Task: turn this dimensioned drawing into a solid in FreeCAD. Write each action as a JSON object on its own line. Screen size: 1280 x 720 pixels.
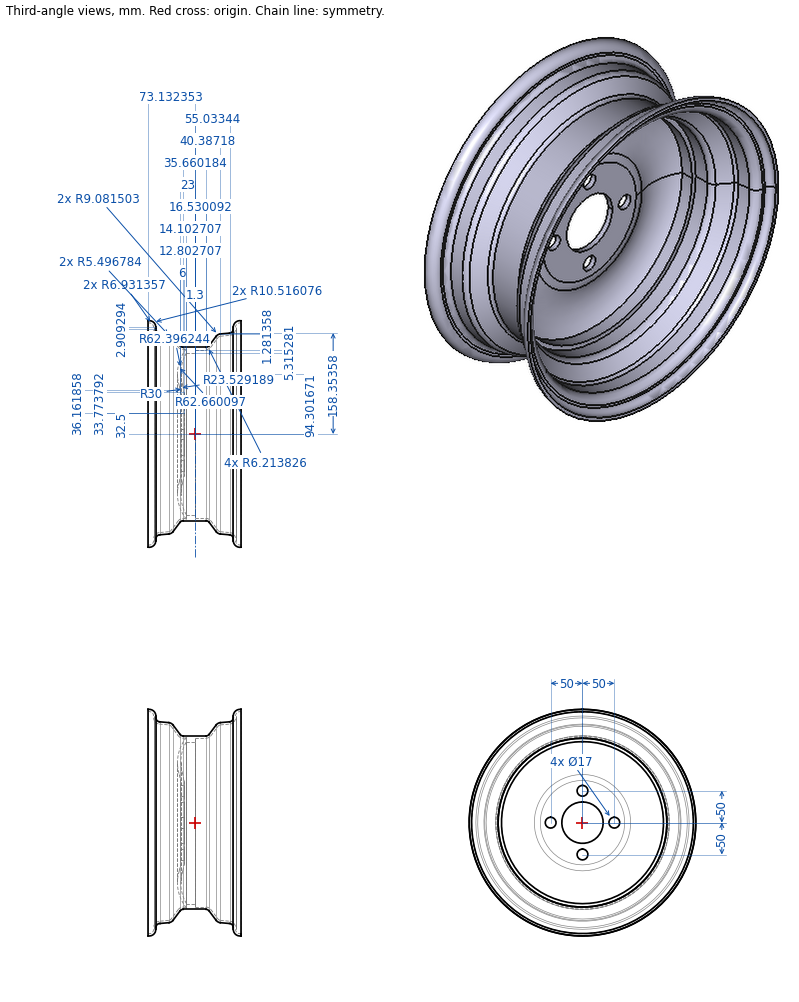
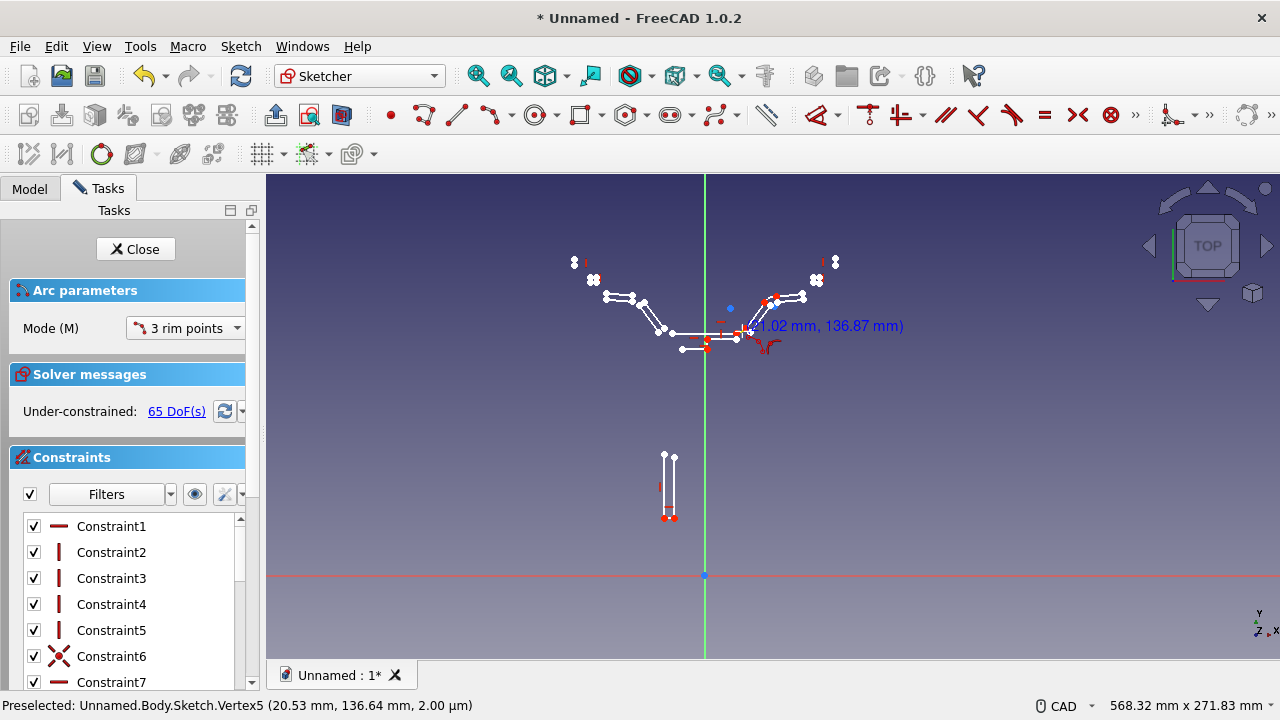
{"action": "scroll", "coordinate": [673, 333], "scroll_direction": "up", "scroll_amount": 3}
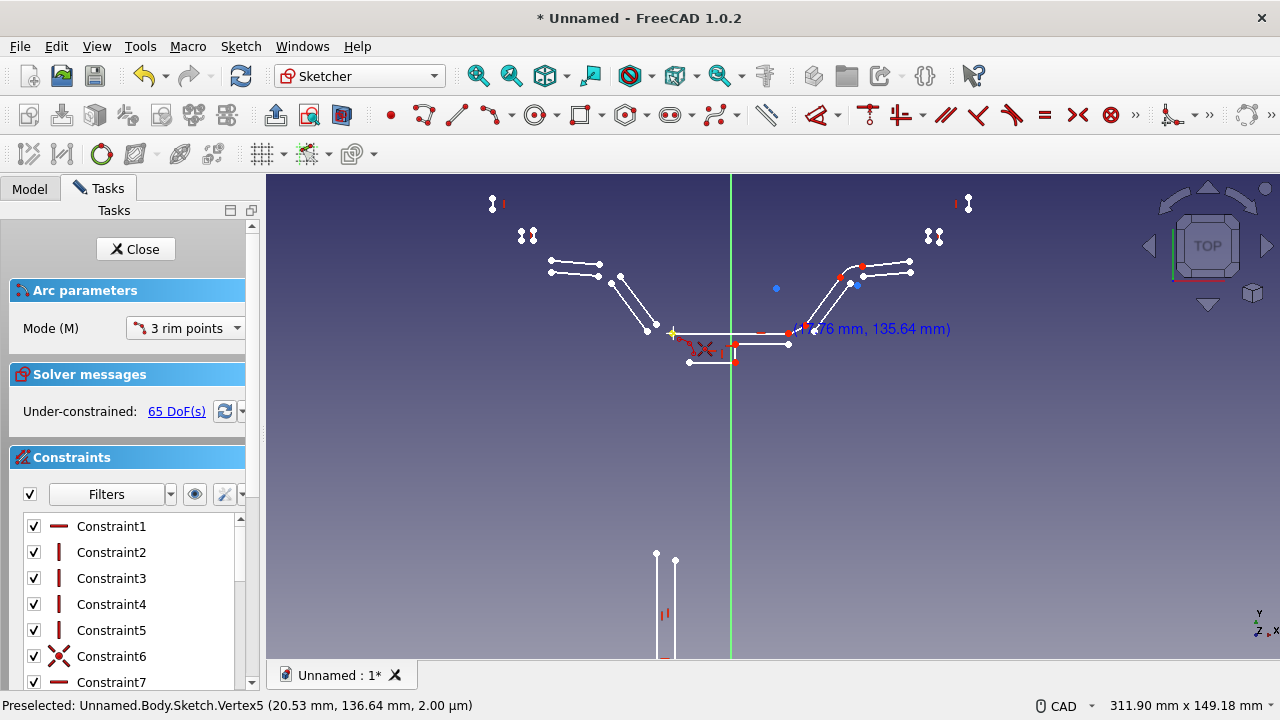
{"action": "left_click", "coordinate": [673, 334]}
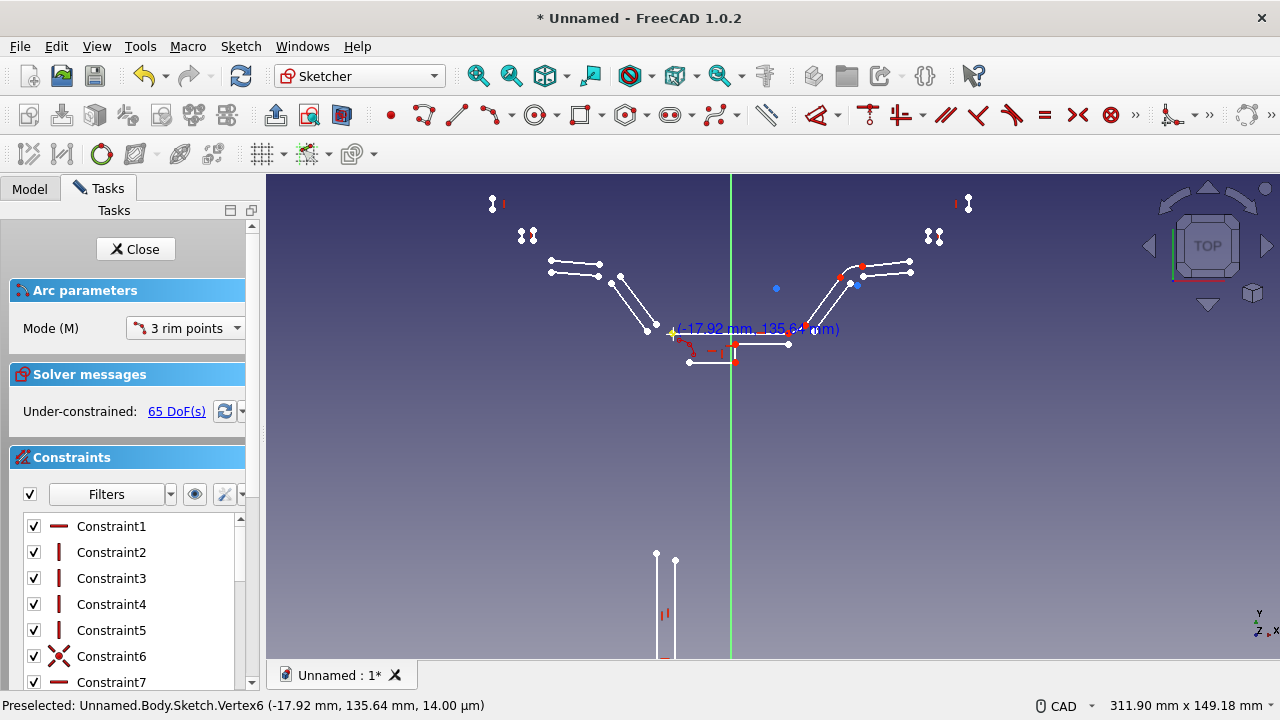
{"action": "scroll", "coordinate": [657, 324], "scroll_direction": "up", "scroll_amount": 2}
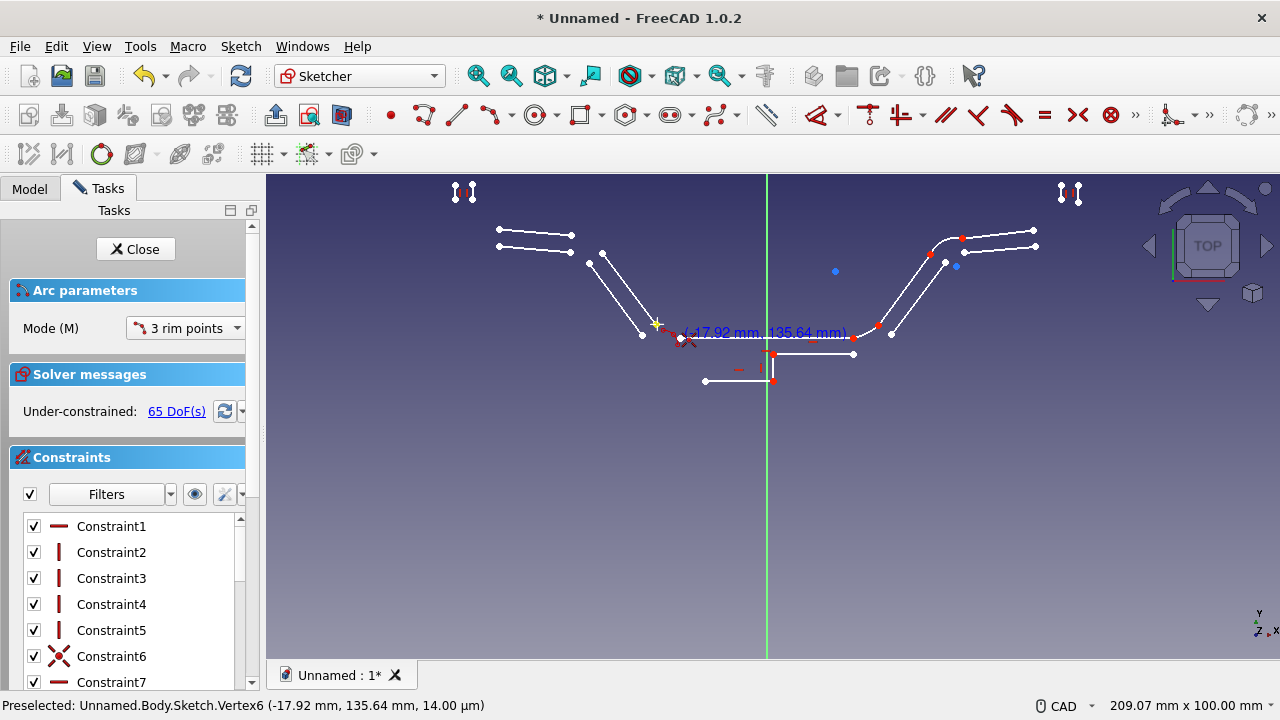
{"action": "left_click", "coordinate": [656, 325]}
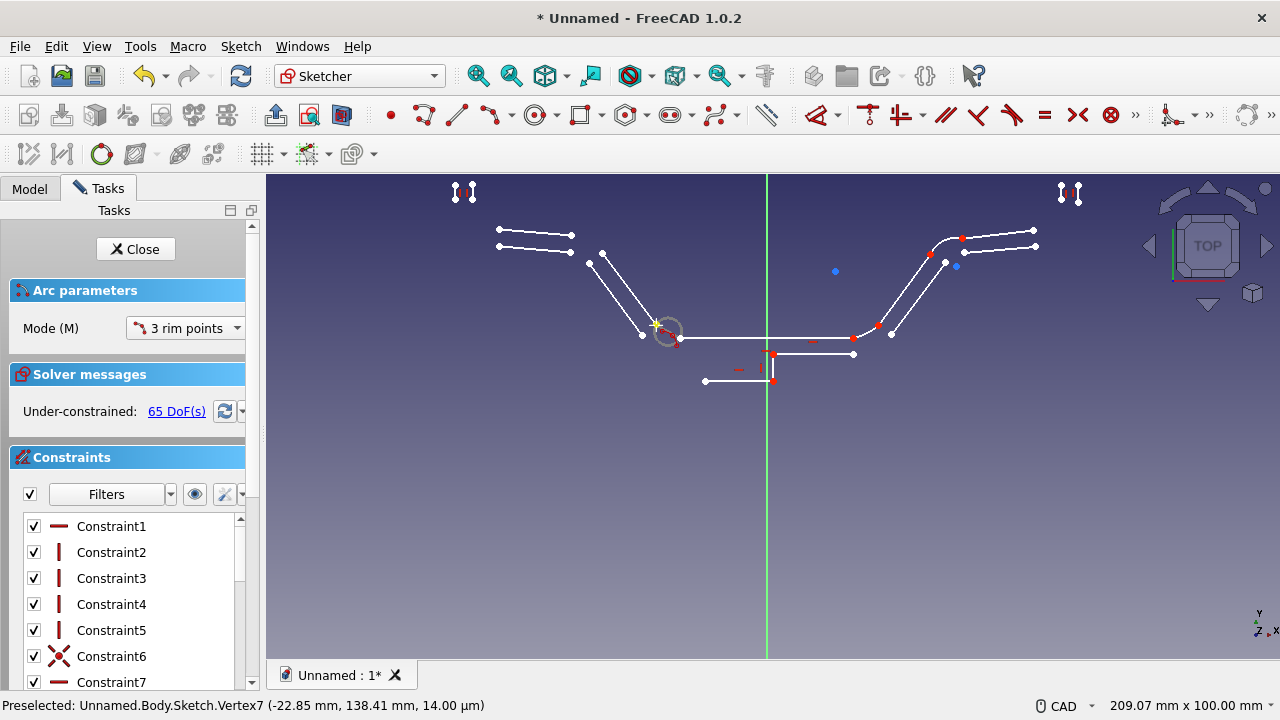
{"action": "scroll", "coordinate": [667, 333], "scroll_direction": "up", "scroll_amount": 9}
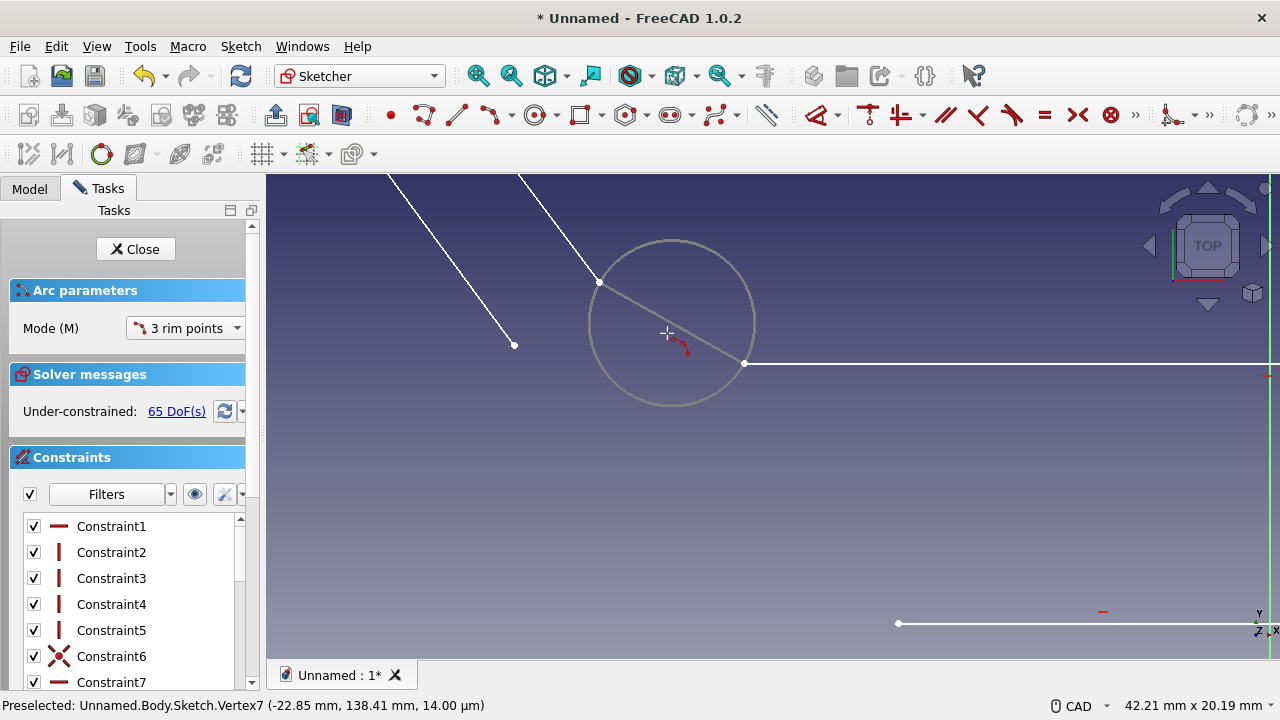
{"action": "left_click", "coordinate": [665, 331]}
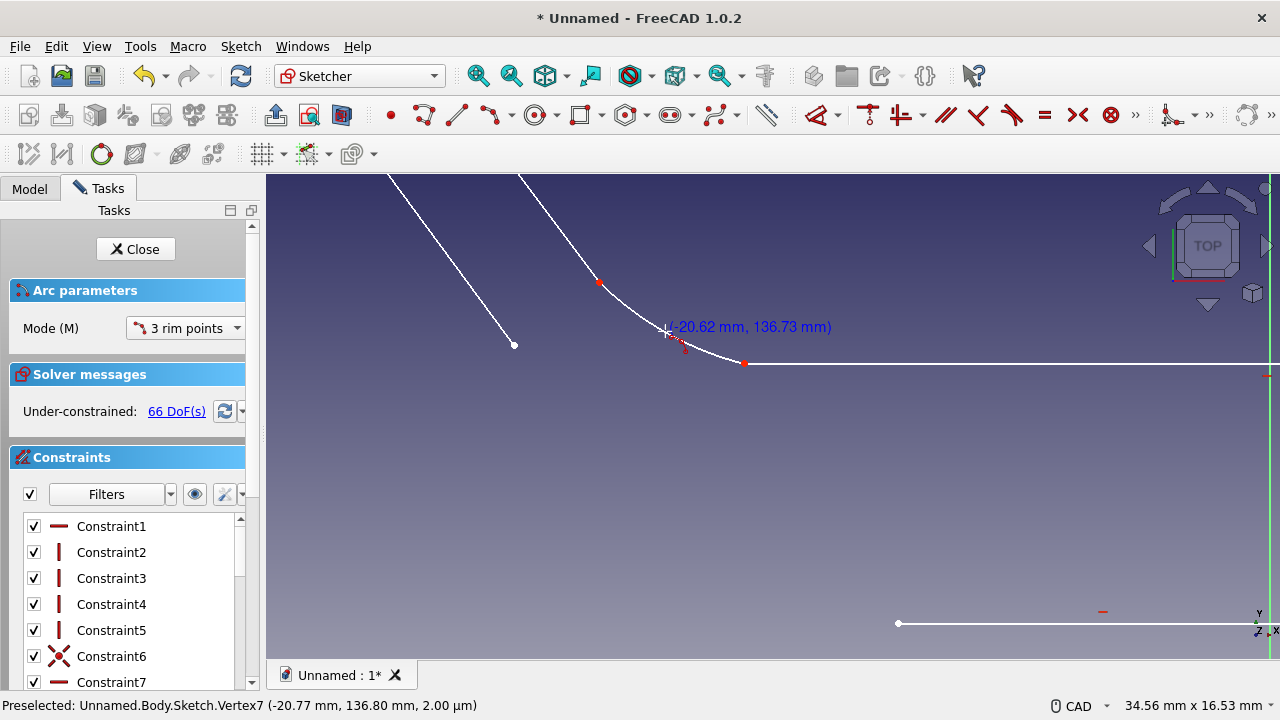
{"action": "scroll", "coordinate": [668, 331], "scroll_direction": "down", "scroll_amount": 14}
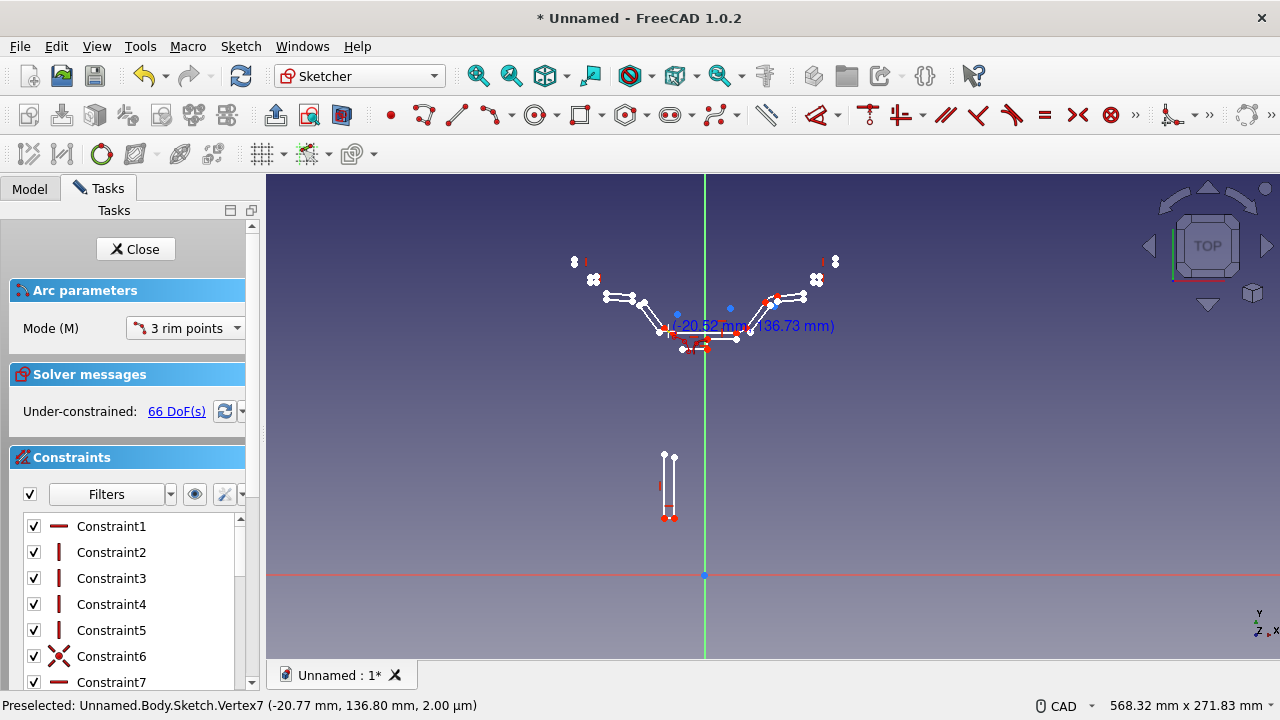
{"action": "scroll", "coordinate": [644, 302], "scroll_direction": "up", "scroll_amount": 5}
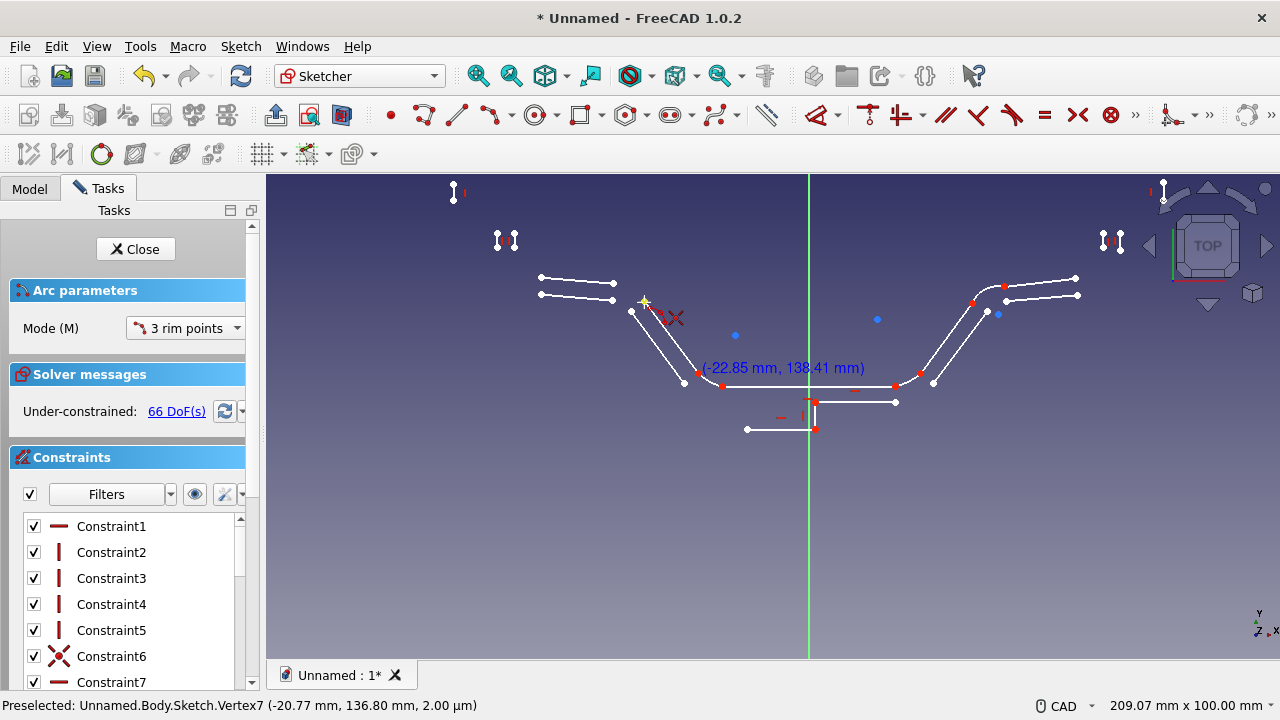
{"action": "left_click", "coordinate": [645, 302]}
{"action": "left_click", "coordinate": [613, 284]}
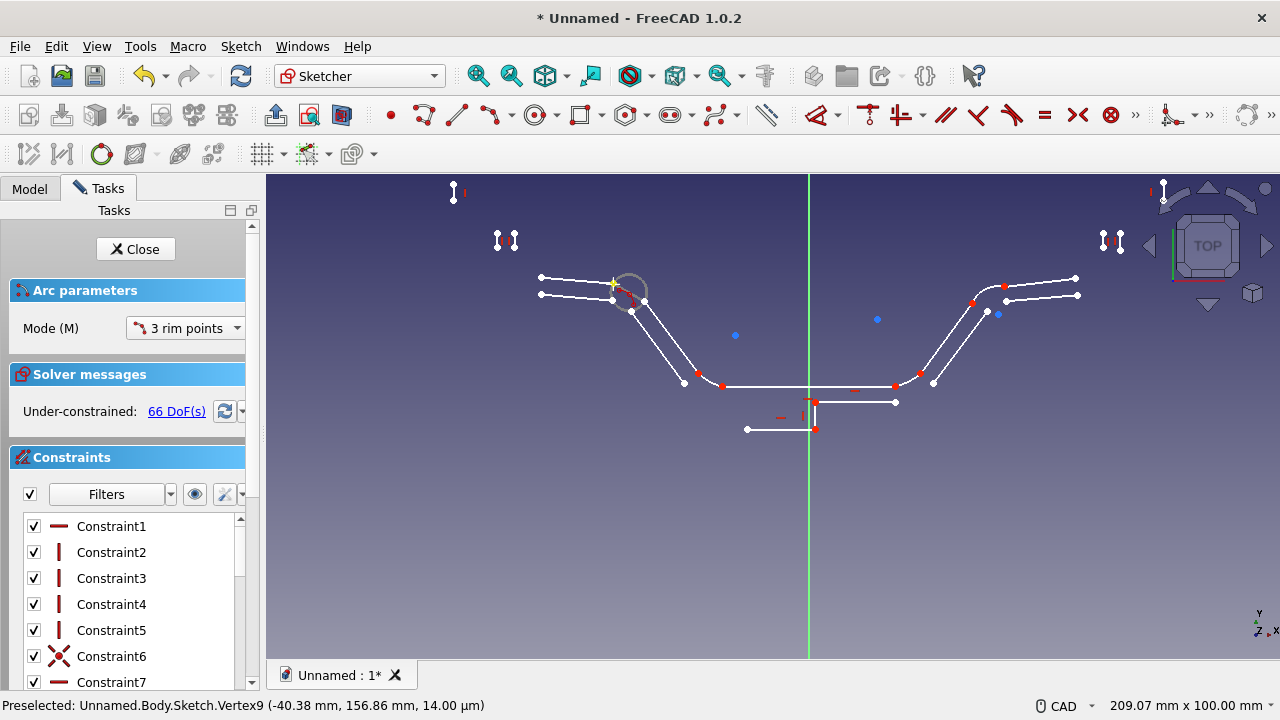
{"action": "scroll", "coordinate": [631, 288], "scroll_direction": "up", "scroll_amount": 8}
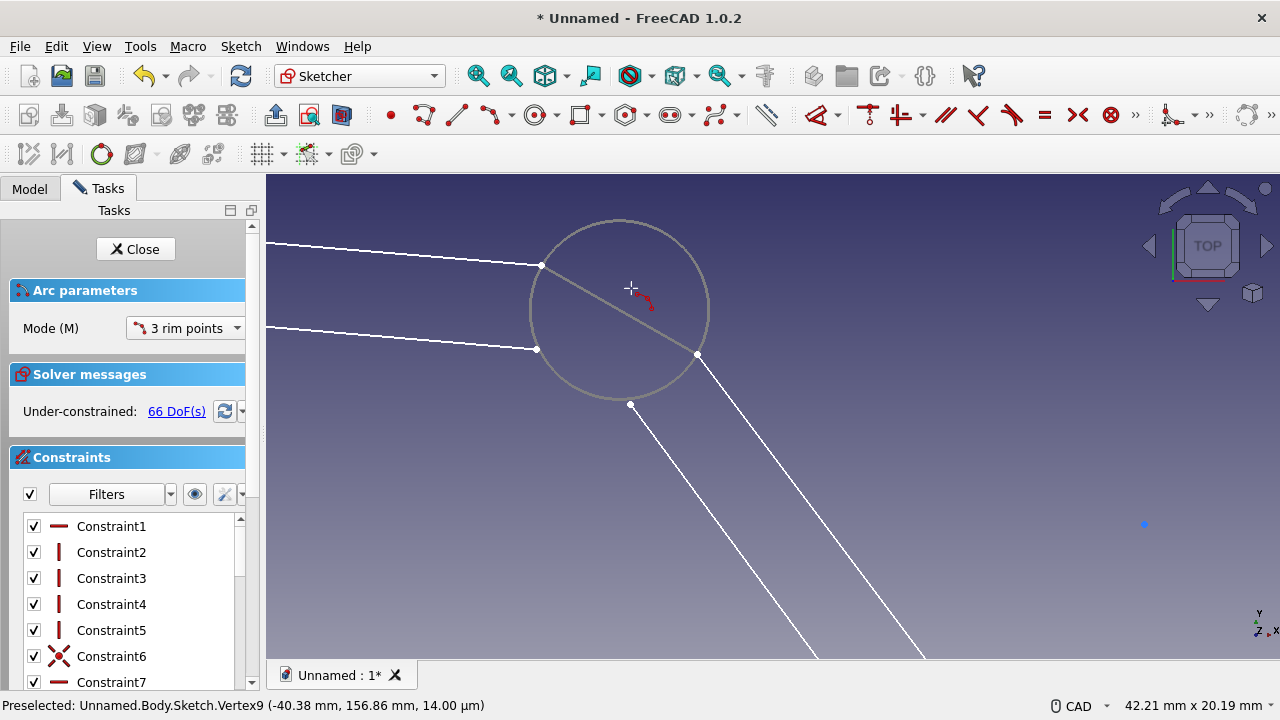
{"action": "left_click", "coordinate": [629, 288]}